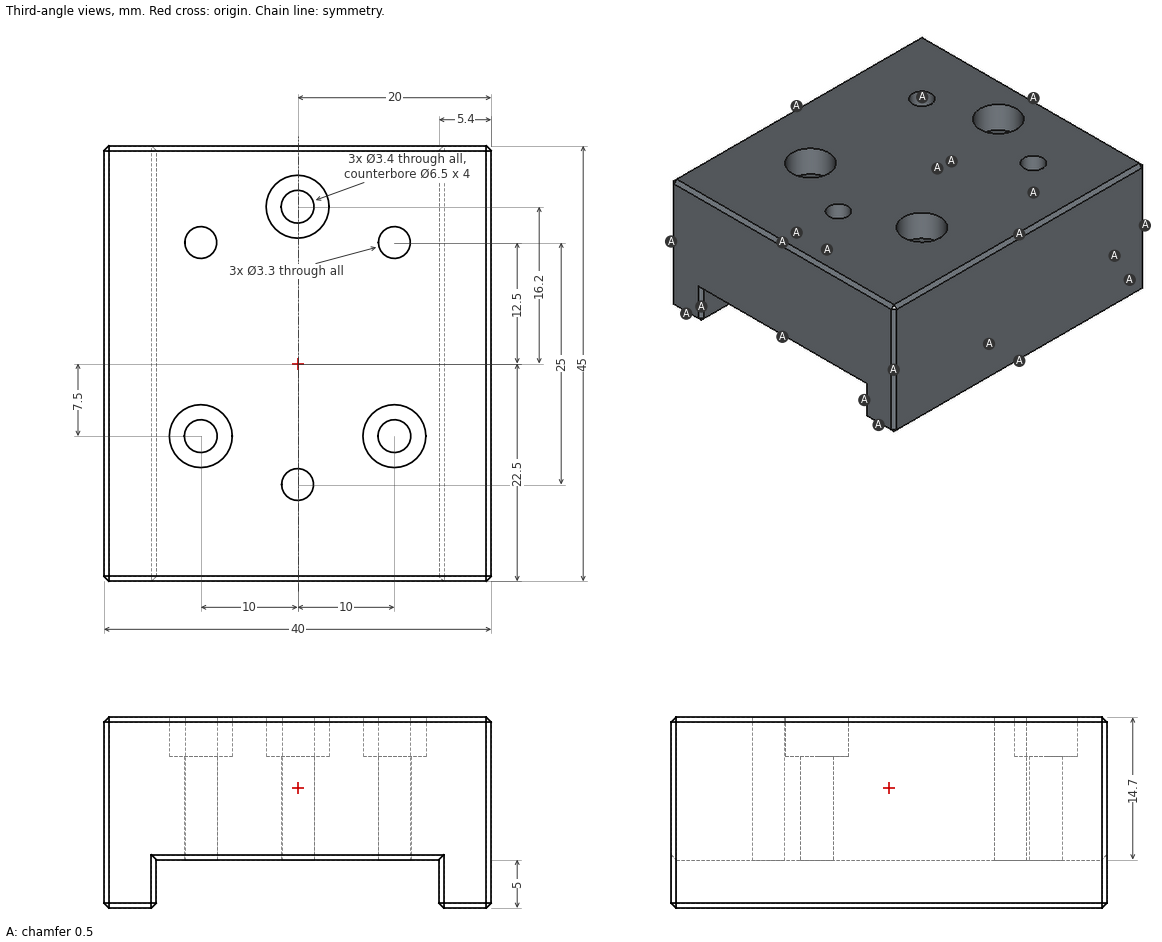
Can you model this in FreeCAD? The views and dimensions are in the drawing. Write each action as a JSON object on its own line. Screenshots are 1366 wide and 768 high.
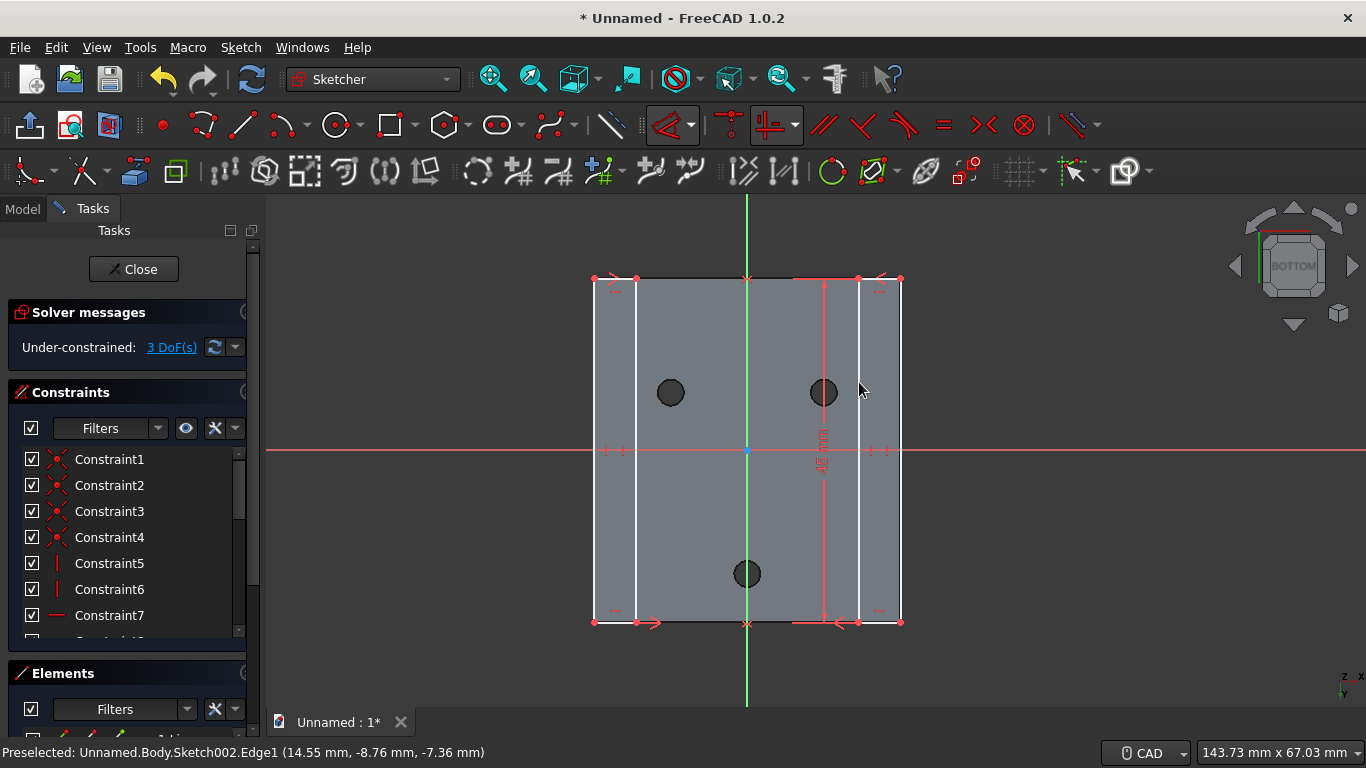
{"action": "left_click", "coordinate": [871, 623]}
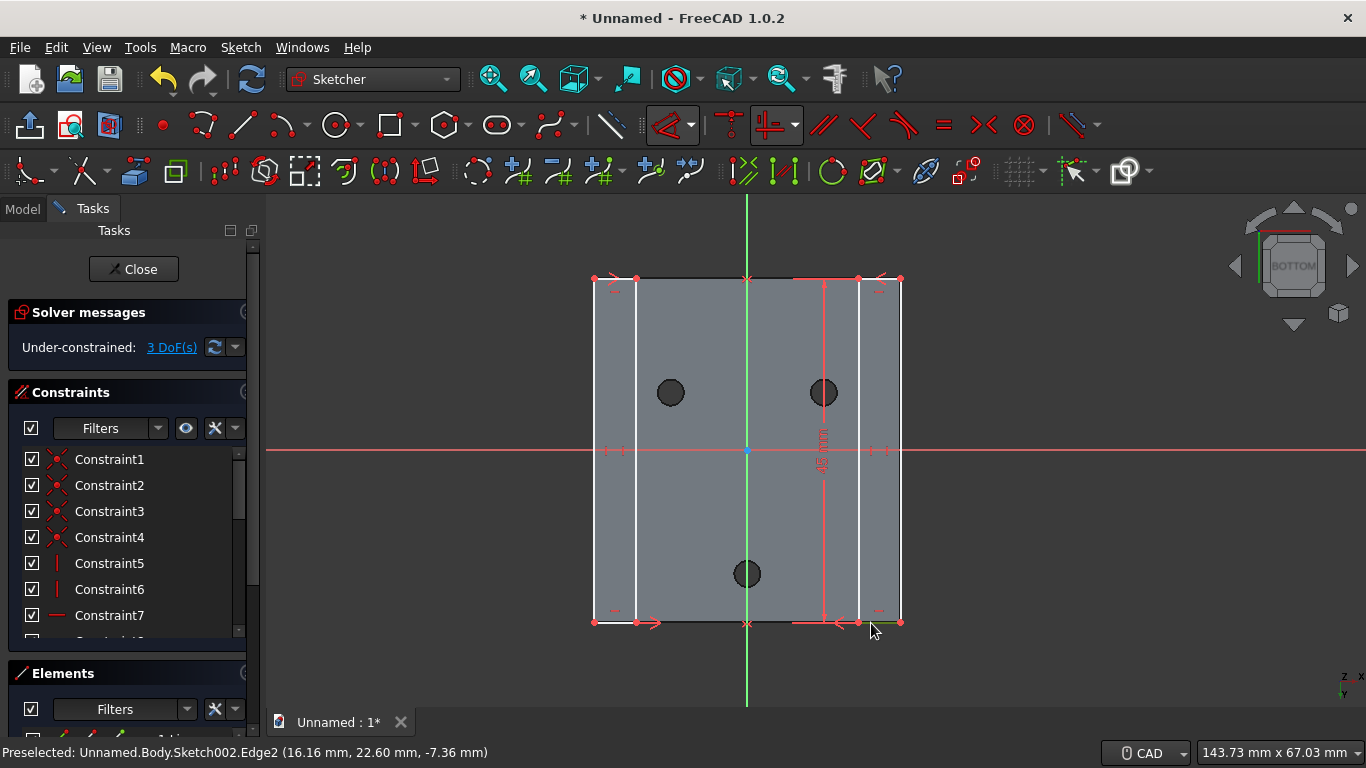
{"action": "key", "text": "l"}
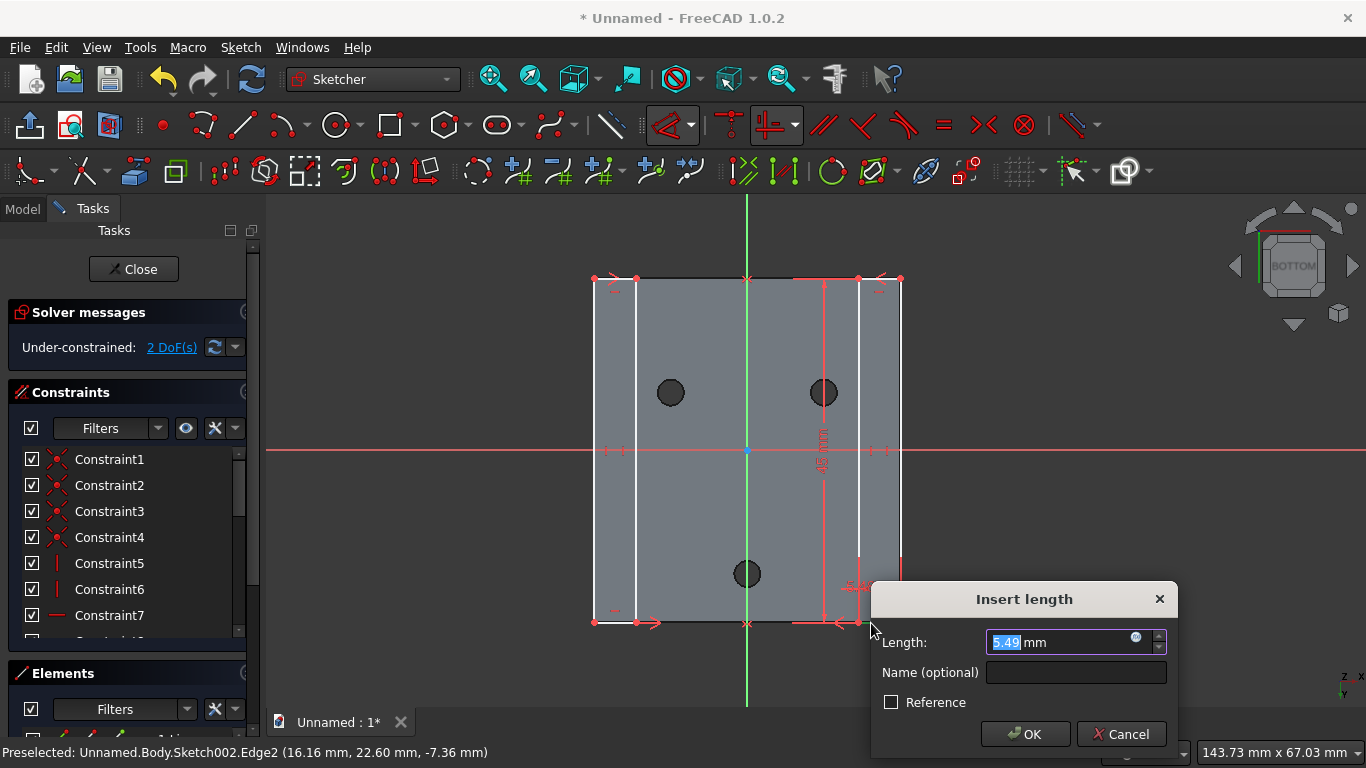
{"action": "type", "text": "5.4"}
{"action": "key", "text": "Return"}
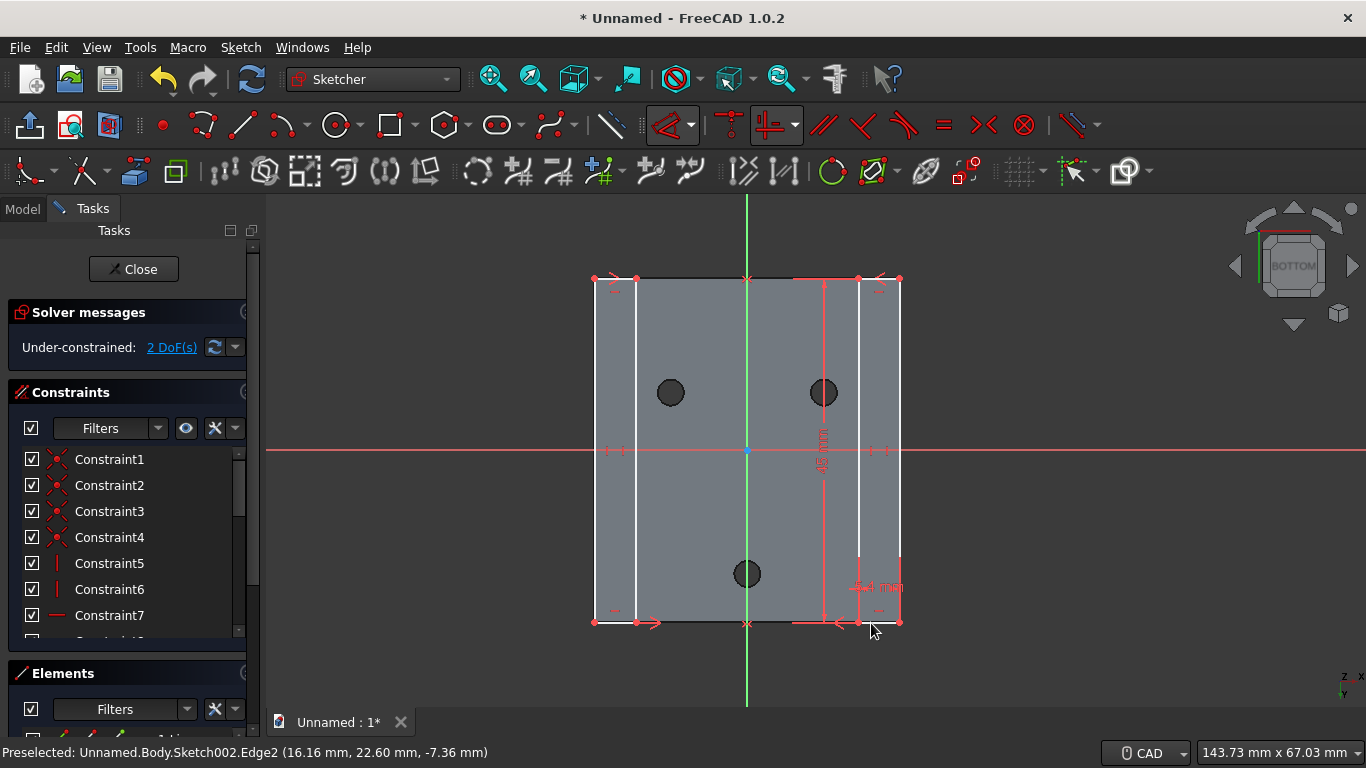
{"action": "left_click", "coordinate": [900, 623]}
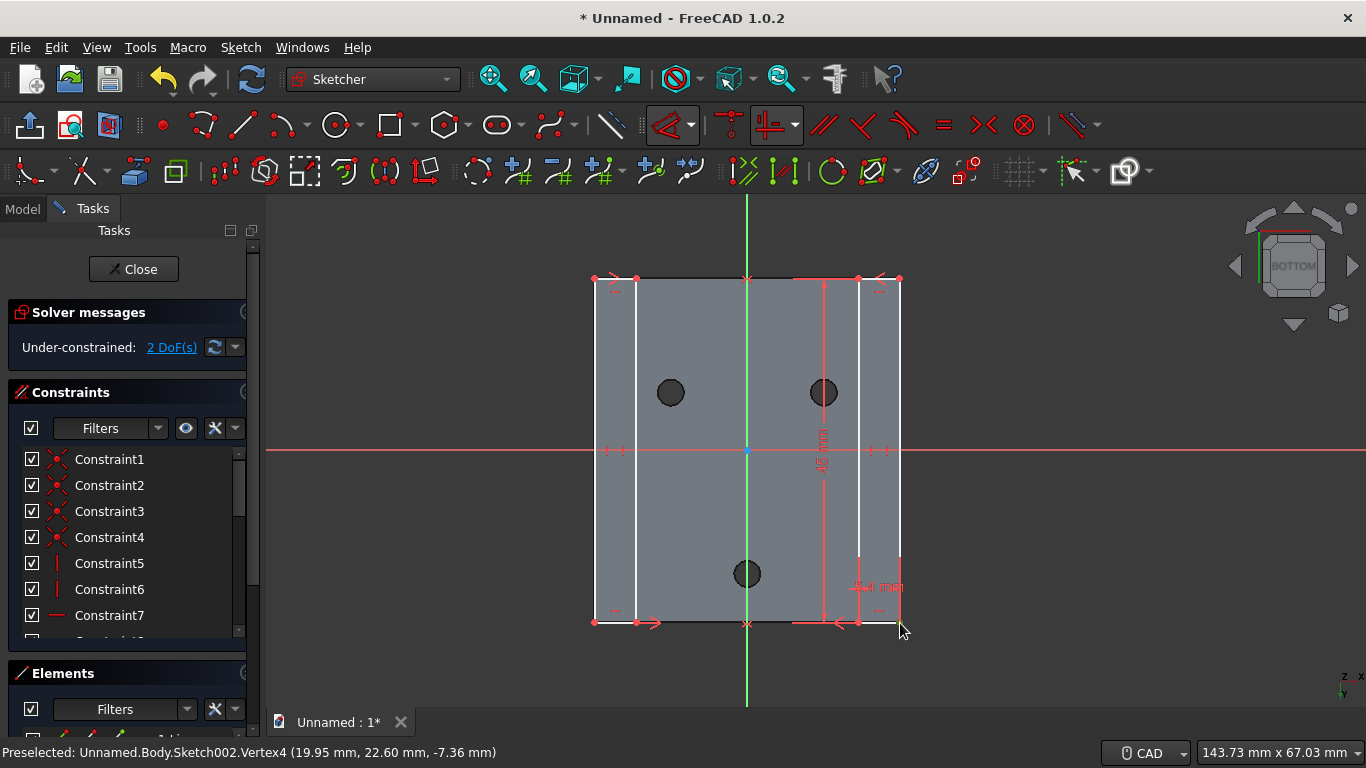
{"action": "left_click", "coordinate": [694, 126]}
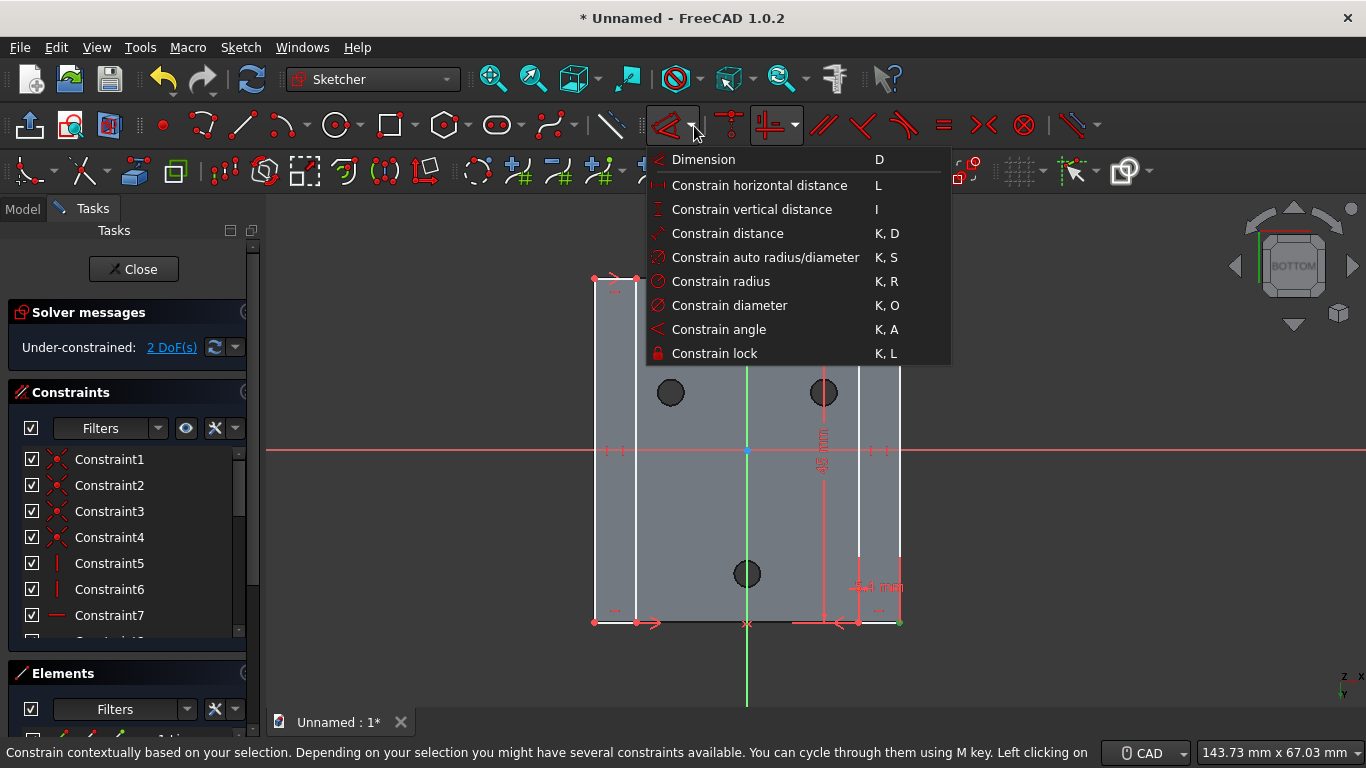
{"action": "left_click", "coordinate": [799, 185]}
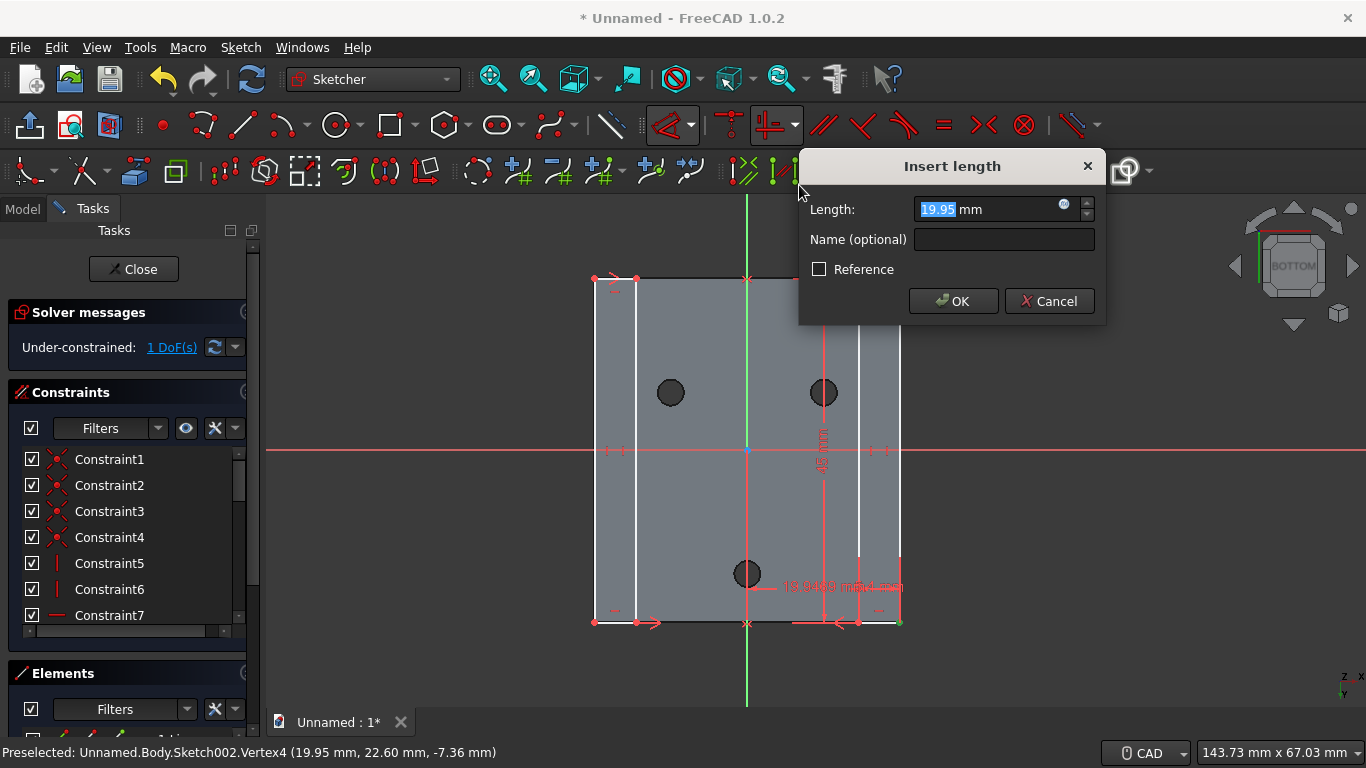
{"action": "type", "text": "20"}
{"action": "key", "text": "Return"}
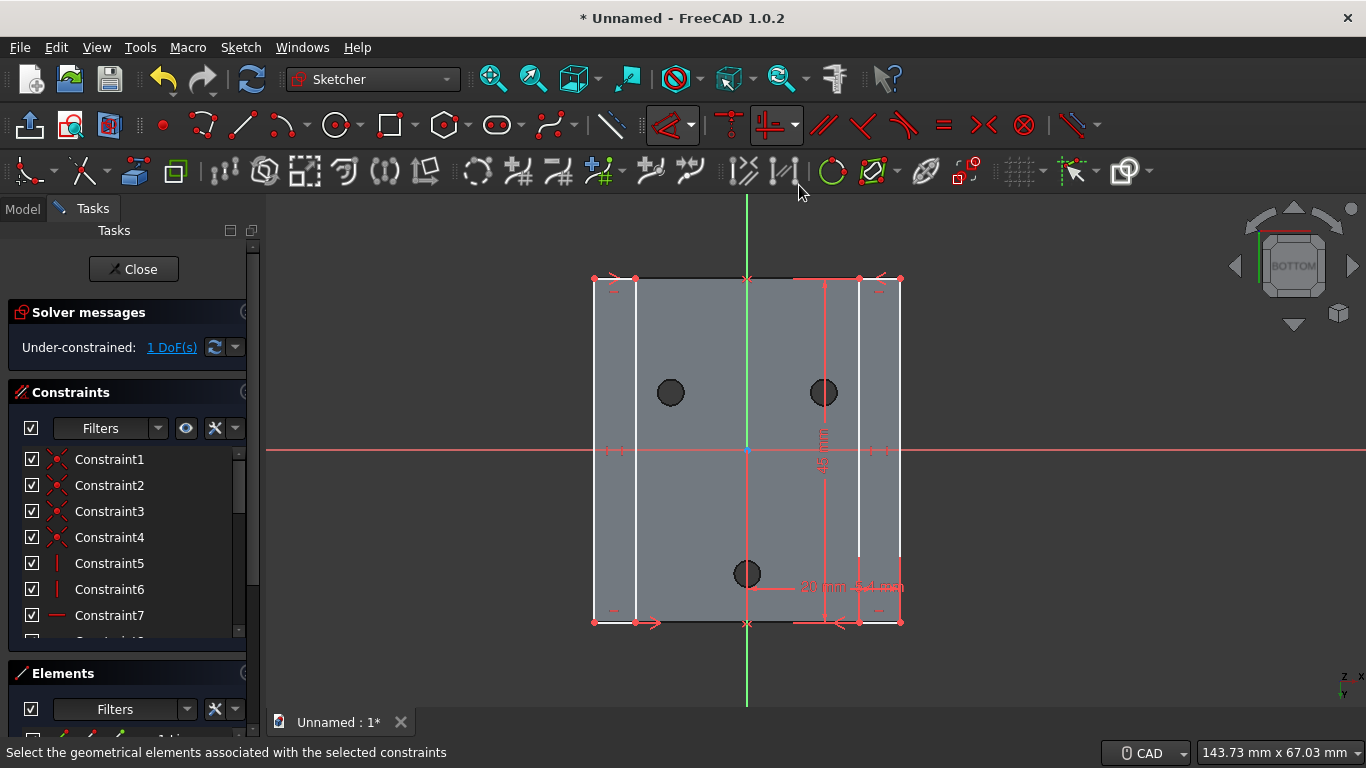
{"action": "left_click", "coordinate": [859, 279]}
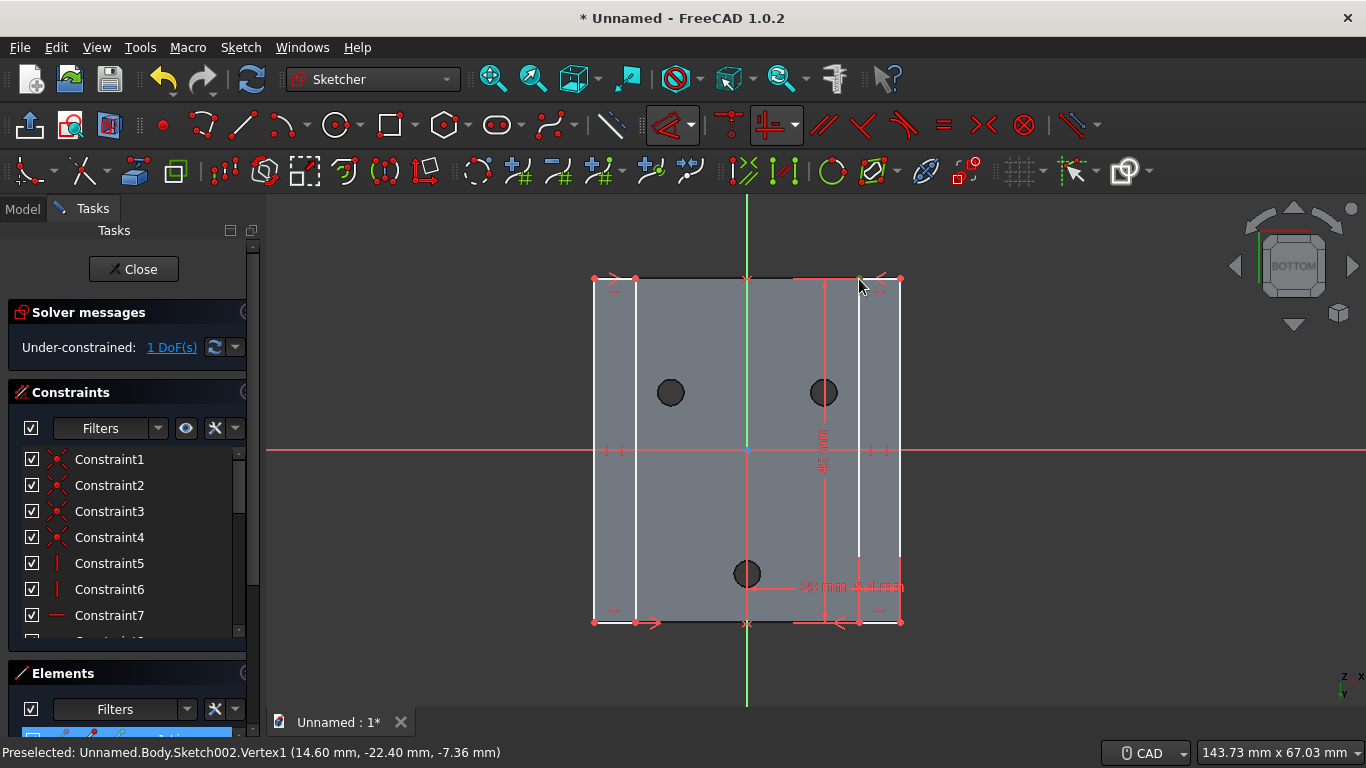
{"action": "key", "text": "i"}